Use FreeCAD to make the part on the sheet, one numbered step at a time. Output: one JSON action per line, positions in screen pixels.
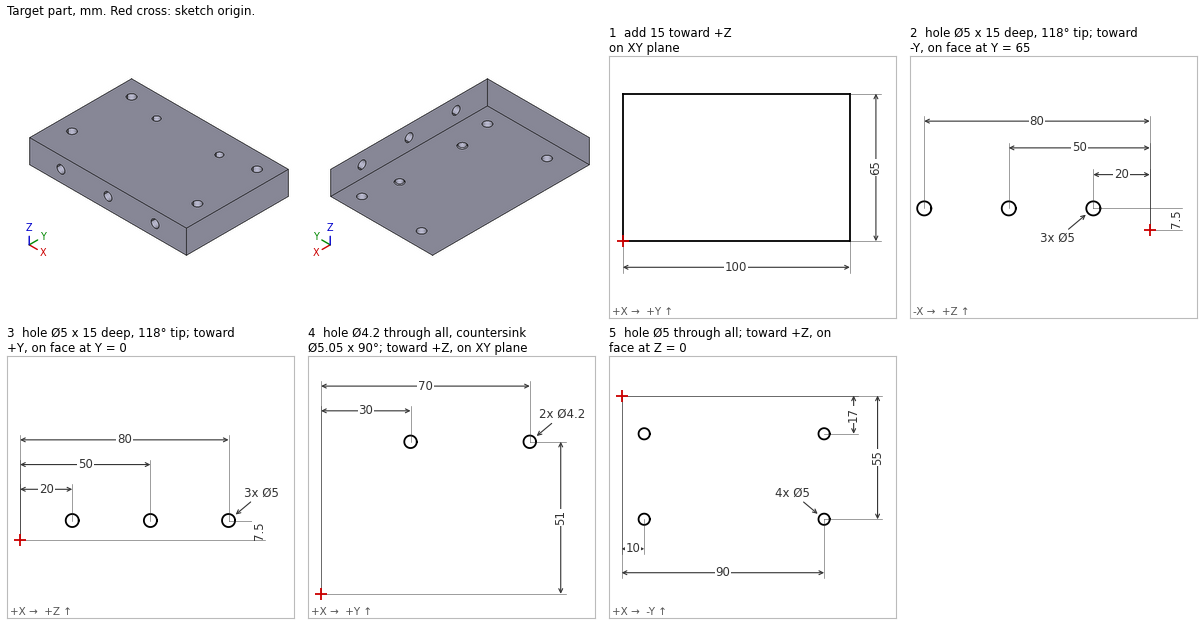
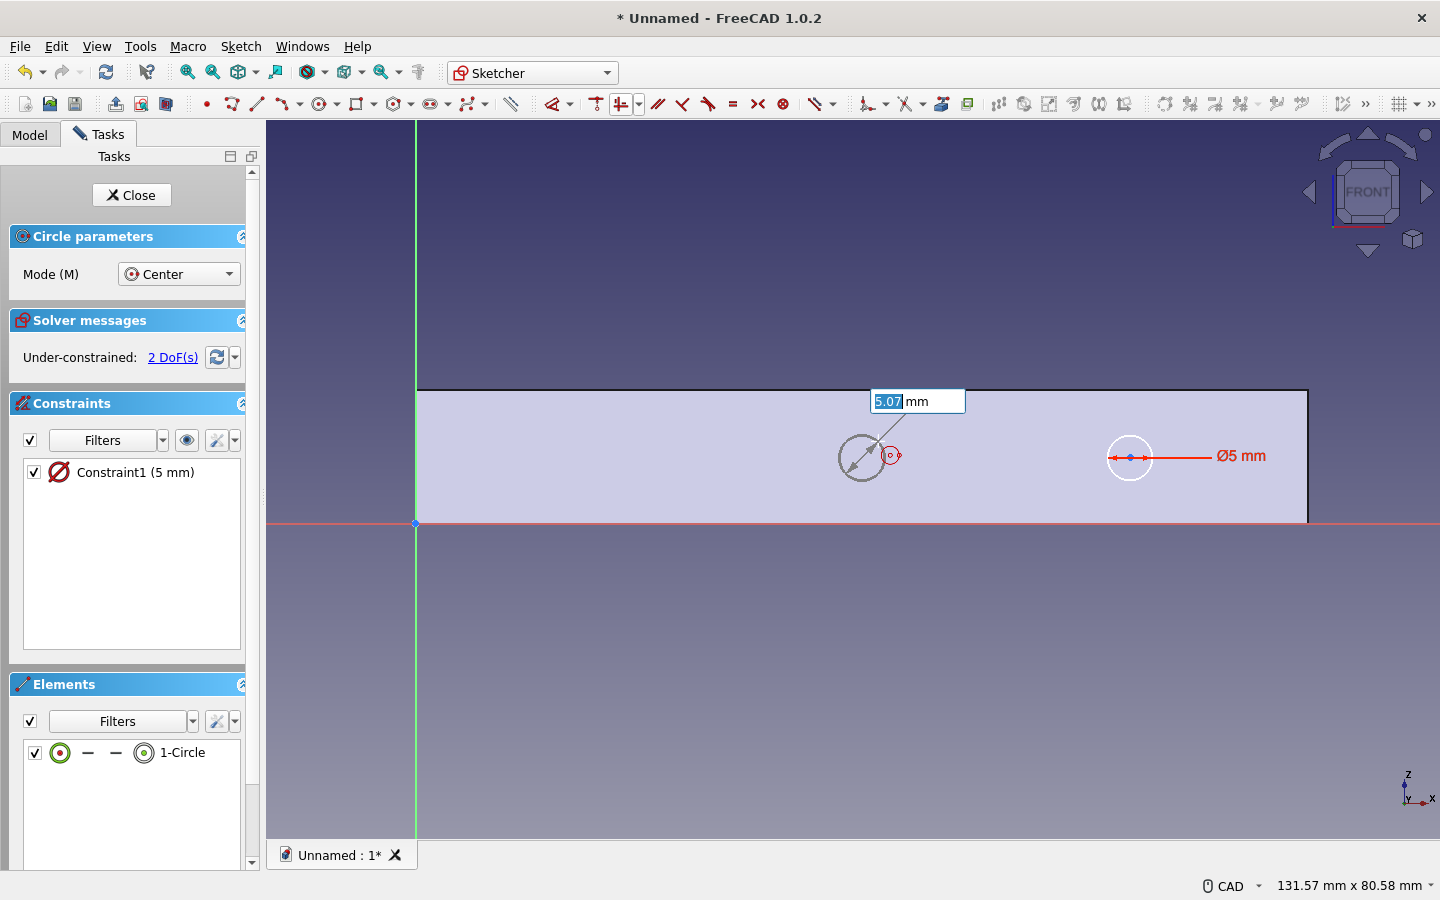
{"action": "type", "text": "5"}
{"action": "key", "text": "Return"}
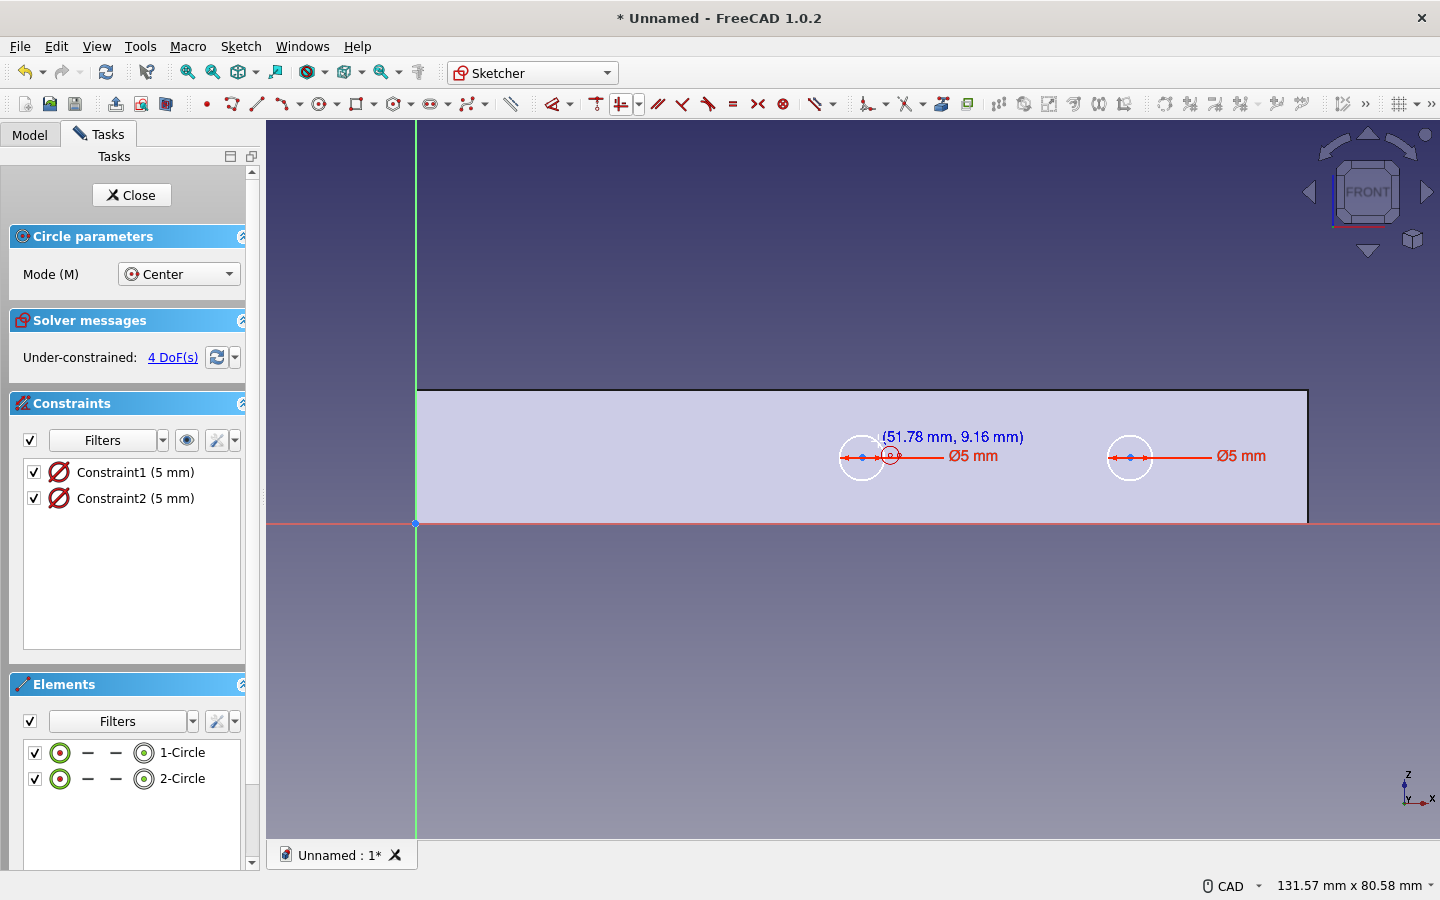
{"action": "left_click", "coordinate": [594, 457]}
{"action": "mouse_move", "coordinate": [610, 441]}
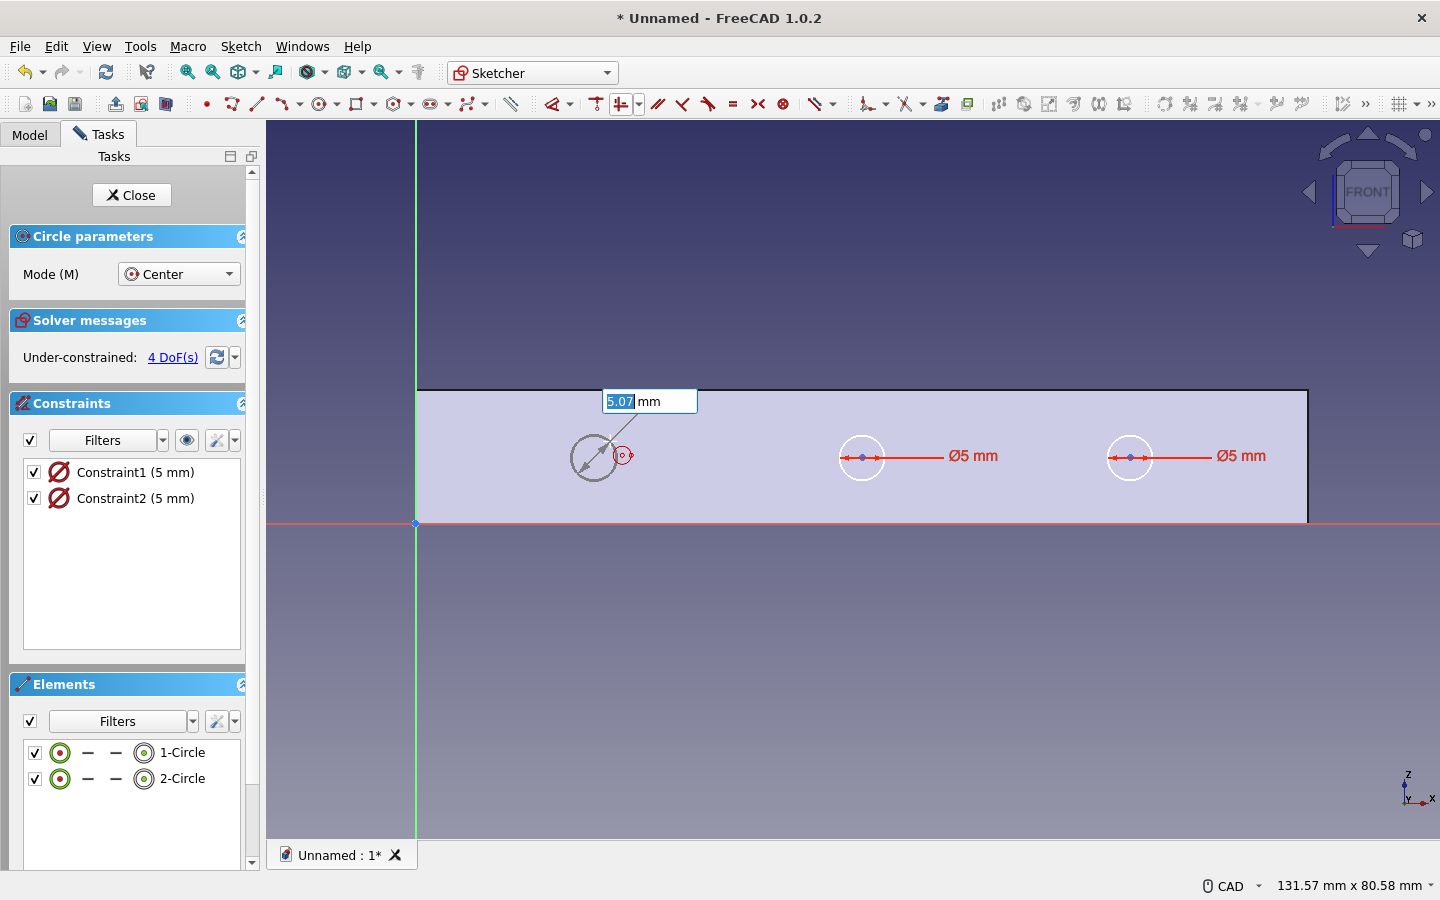
{"action": "type", "text": "5"}
{"action": "key", "text": "Return"}
{"action": "key", "text": "Escape"}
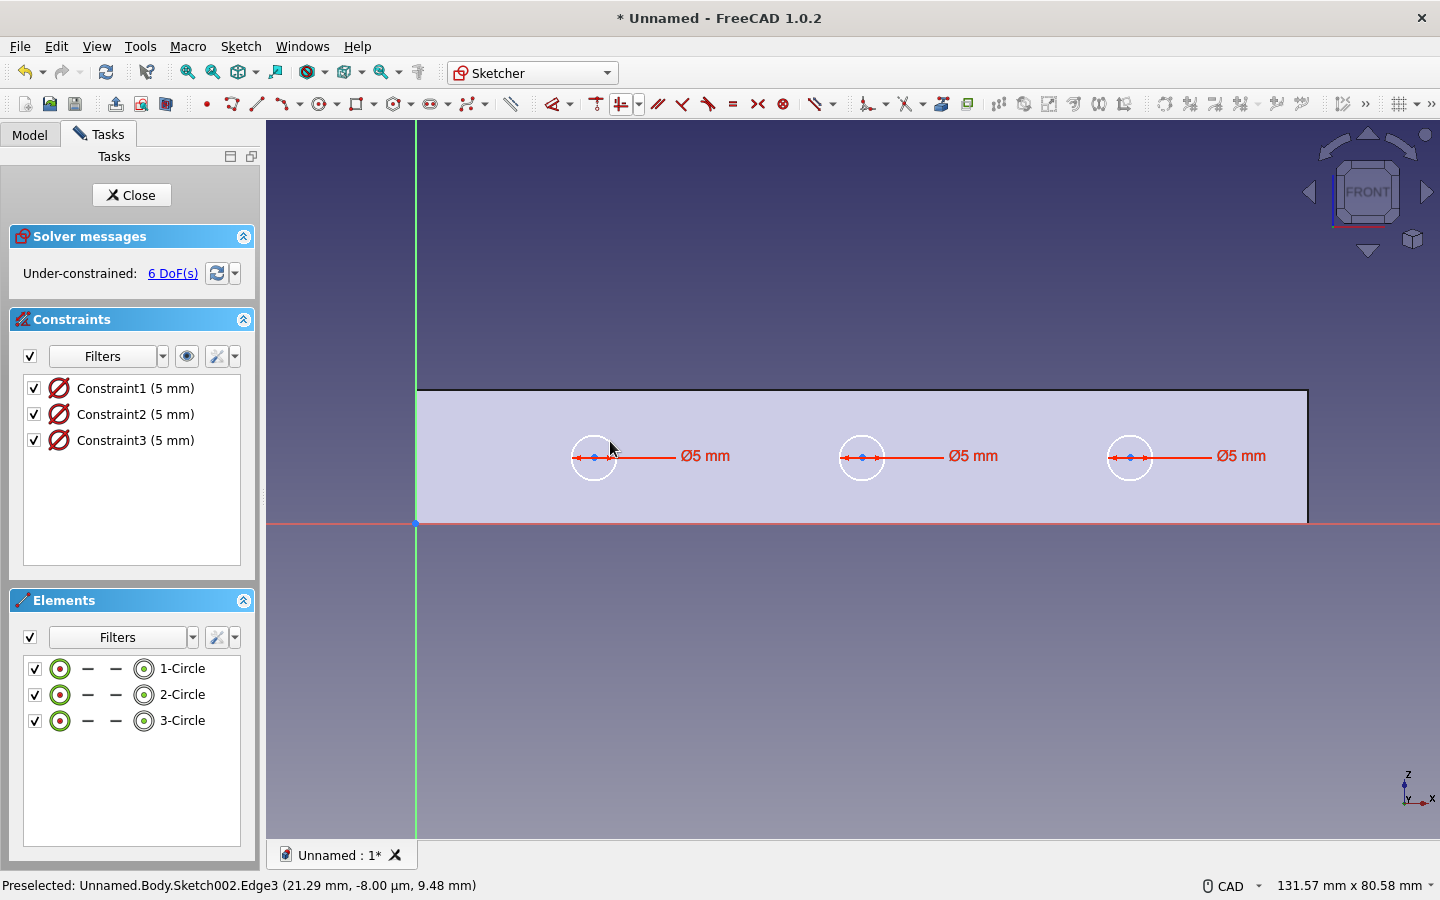
{"action": "left_click", "coordinate": [1130, 458]}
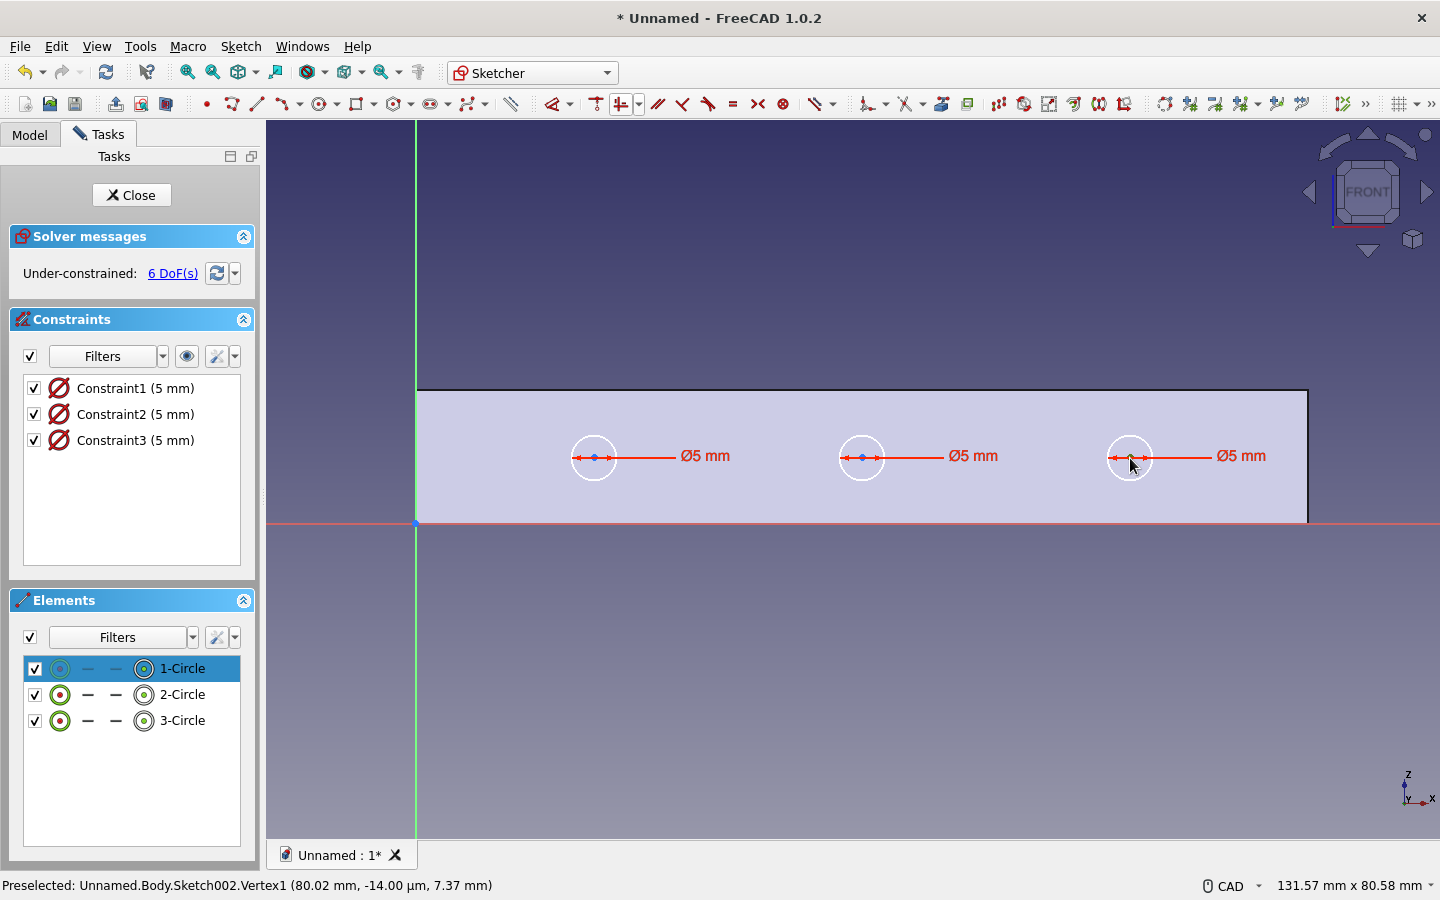
{"action": "left_click", "coordinate": [862, 458]}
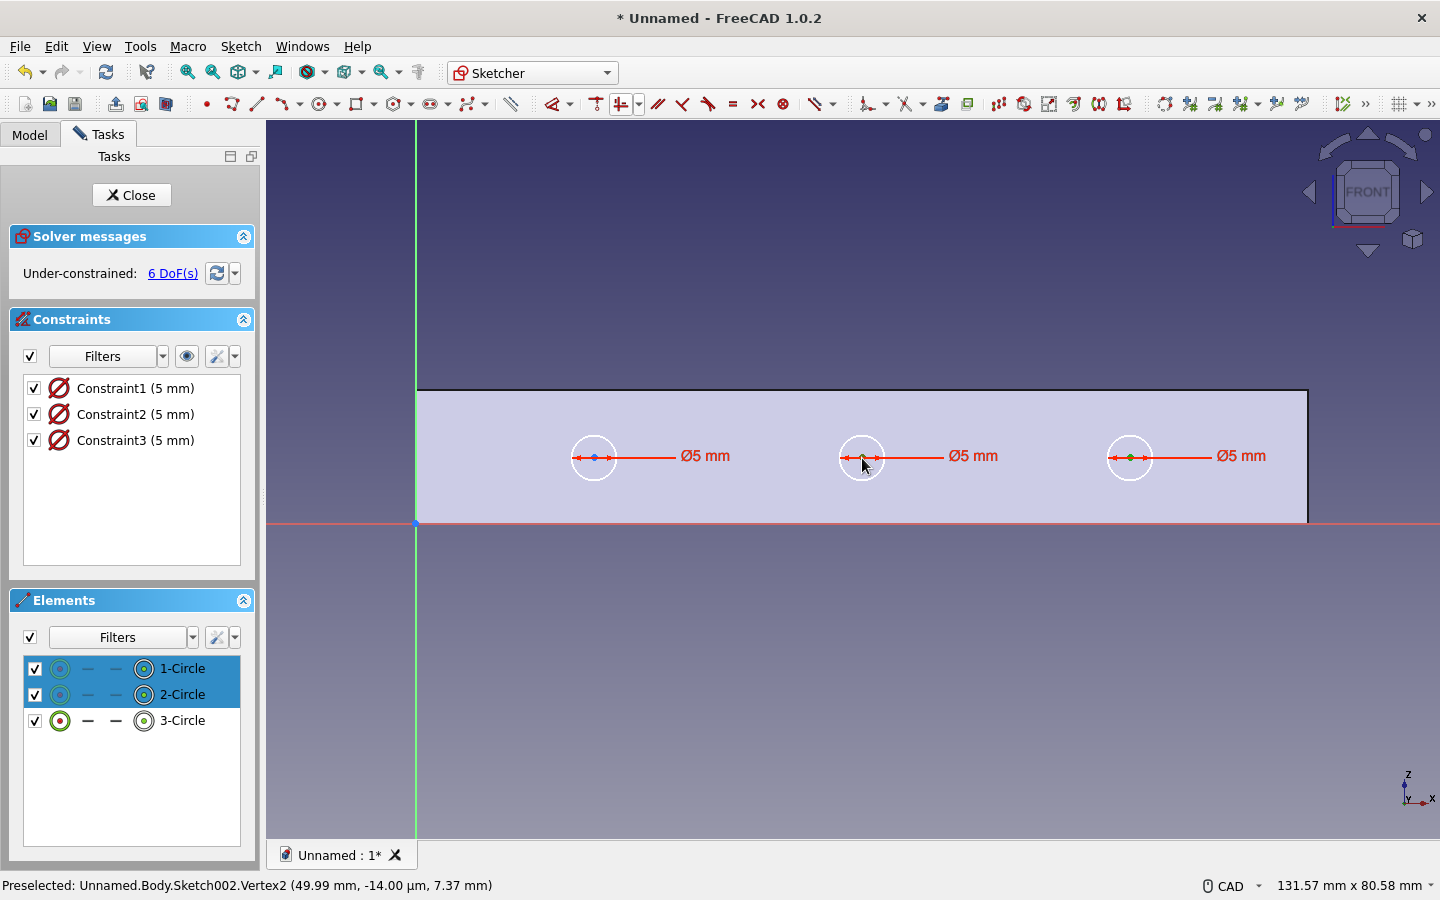
{"action": "left_click", "coordinate": [638, 104]}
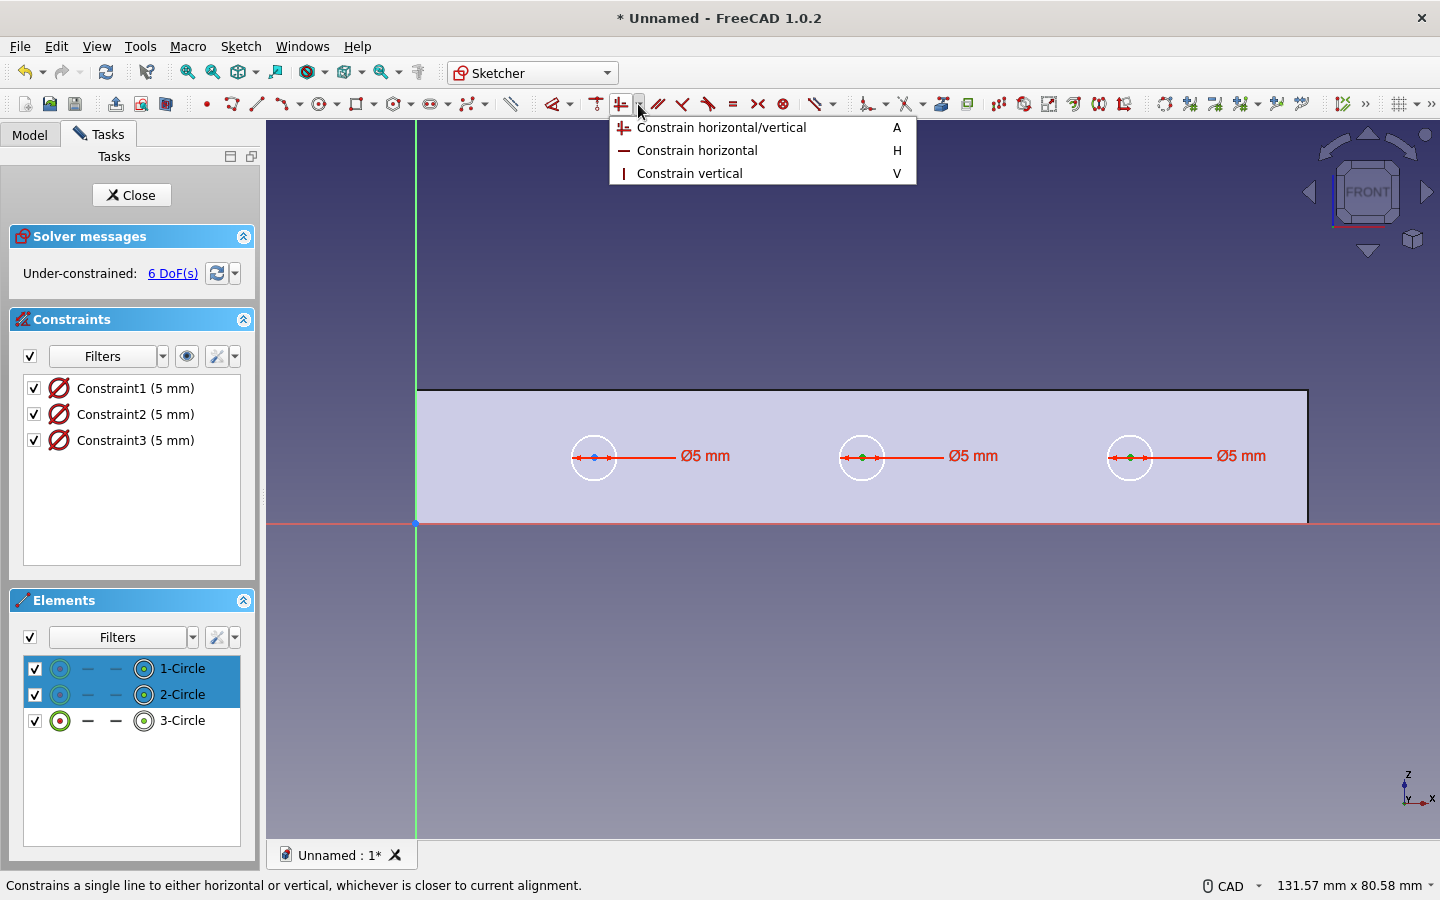
{"action": "left_click", "coordinate": [763, 150]}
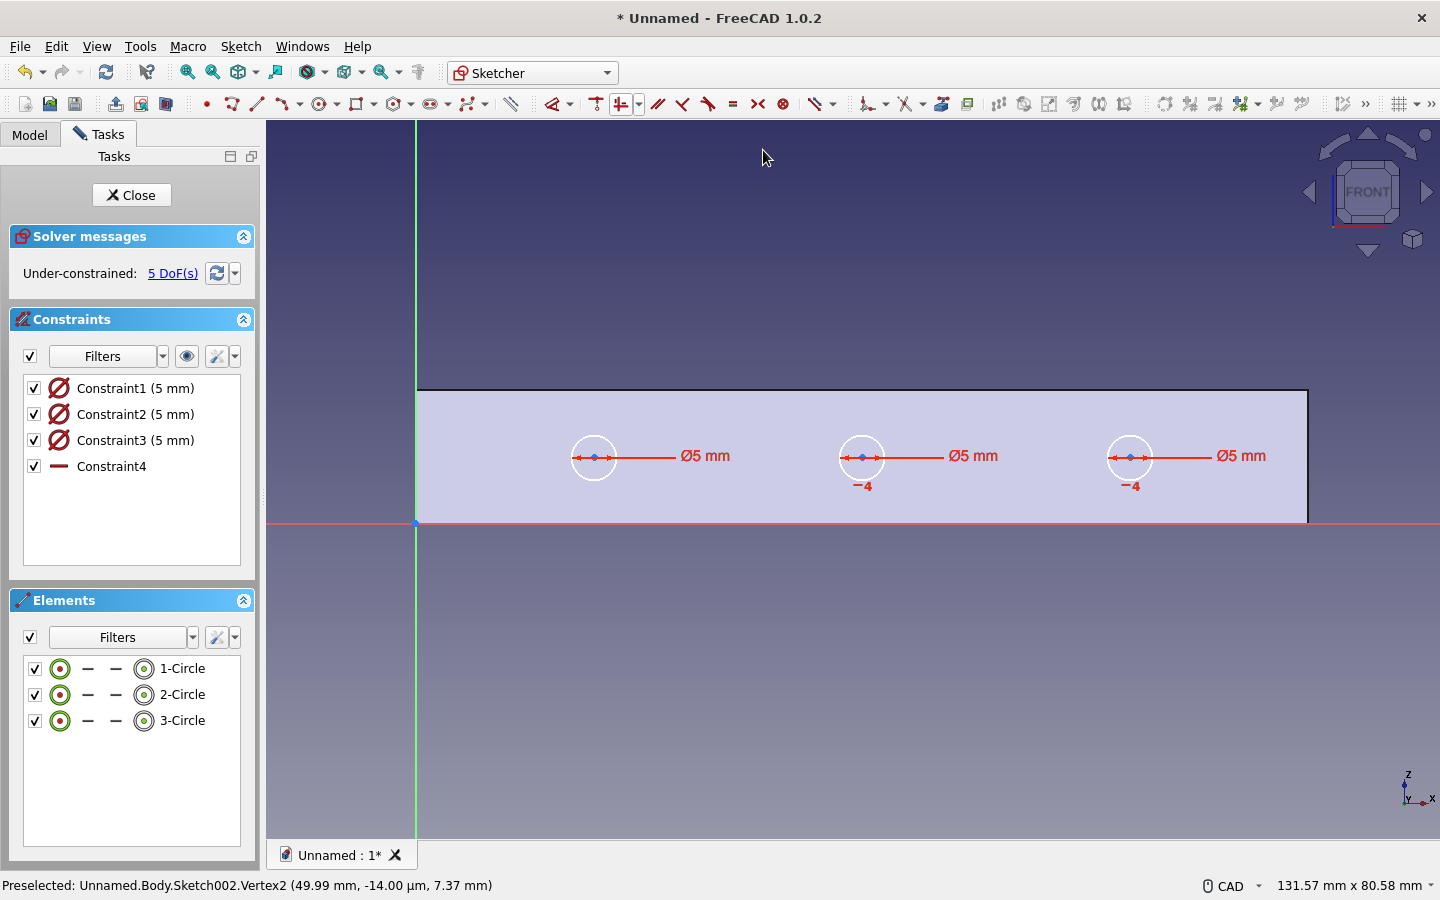
{"action": "left_click", "coordinate": [862, 458]}